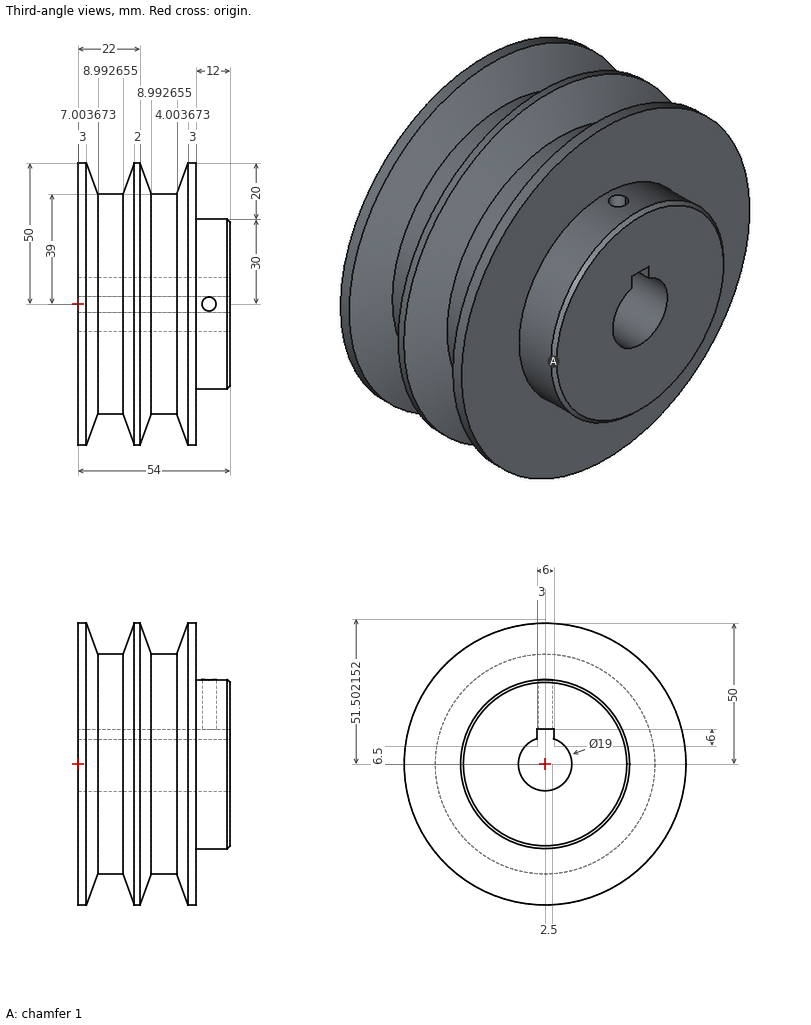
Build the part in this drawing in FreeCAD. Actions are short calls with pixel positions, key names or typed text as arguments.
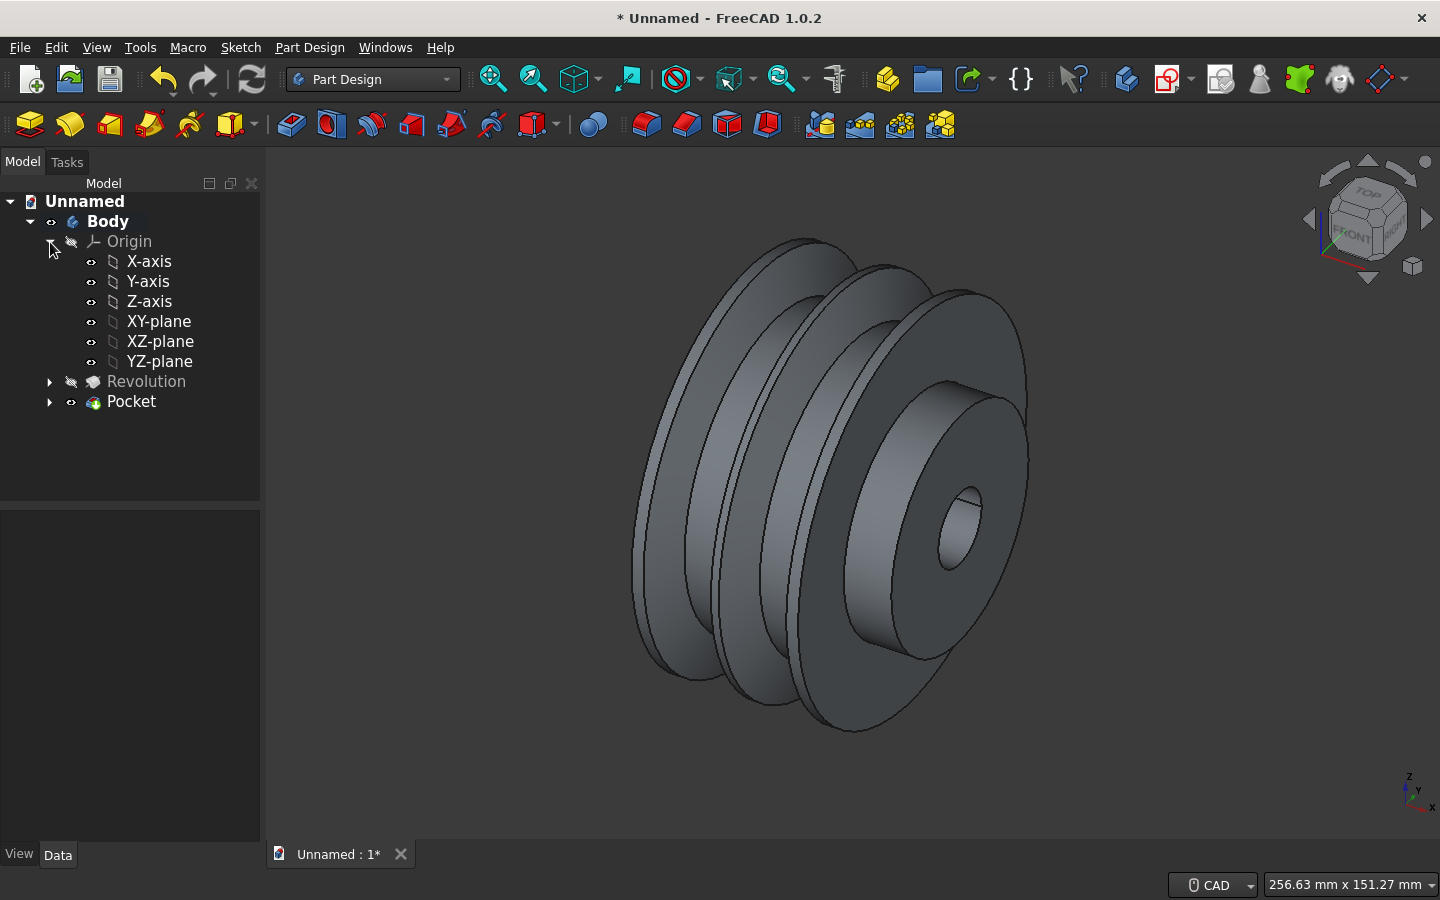
click(136, 362)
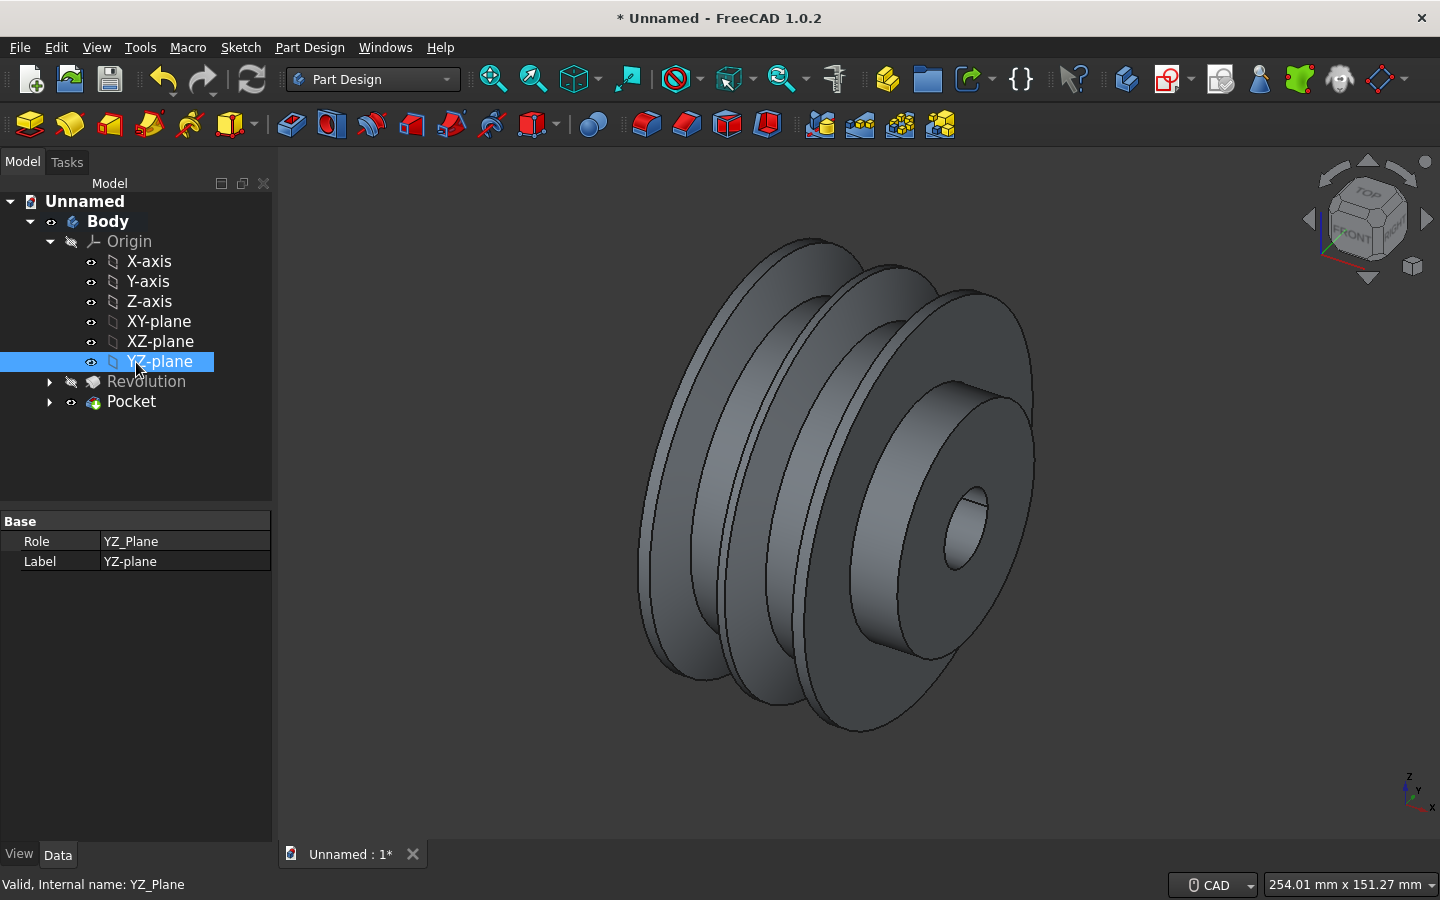
click(1380, 80)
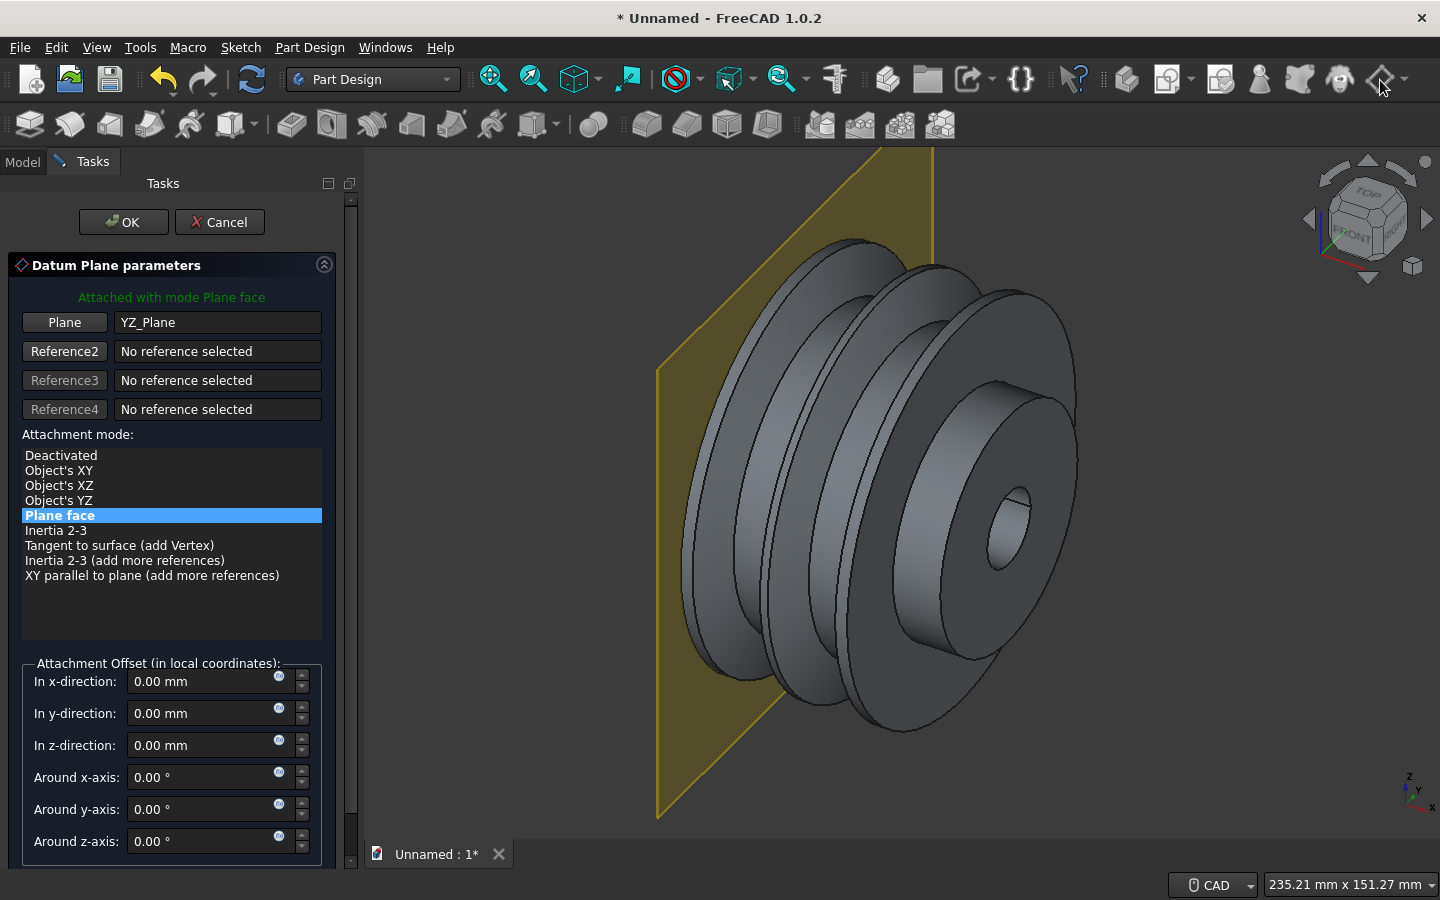
triple_click(210, 745)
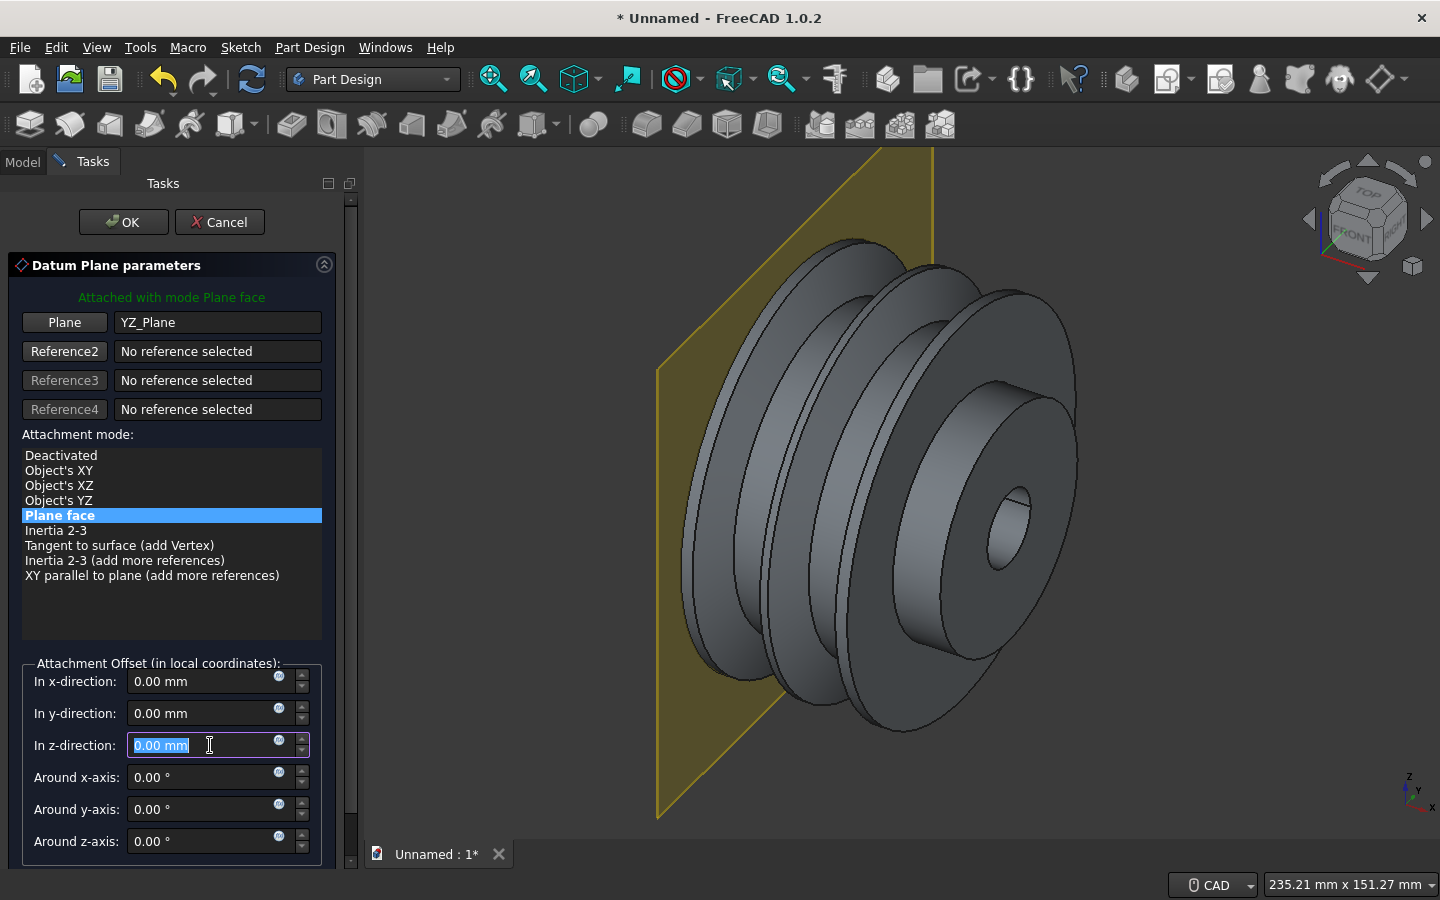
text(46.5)
key(Tab)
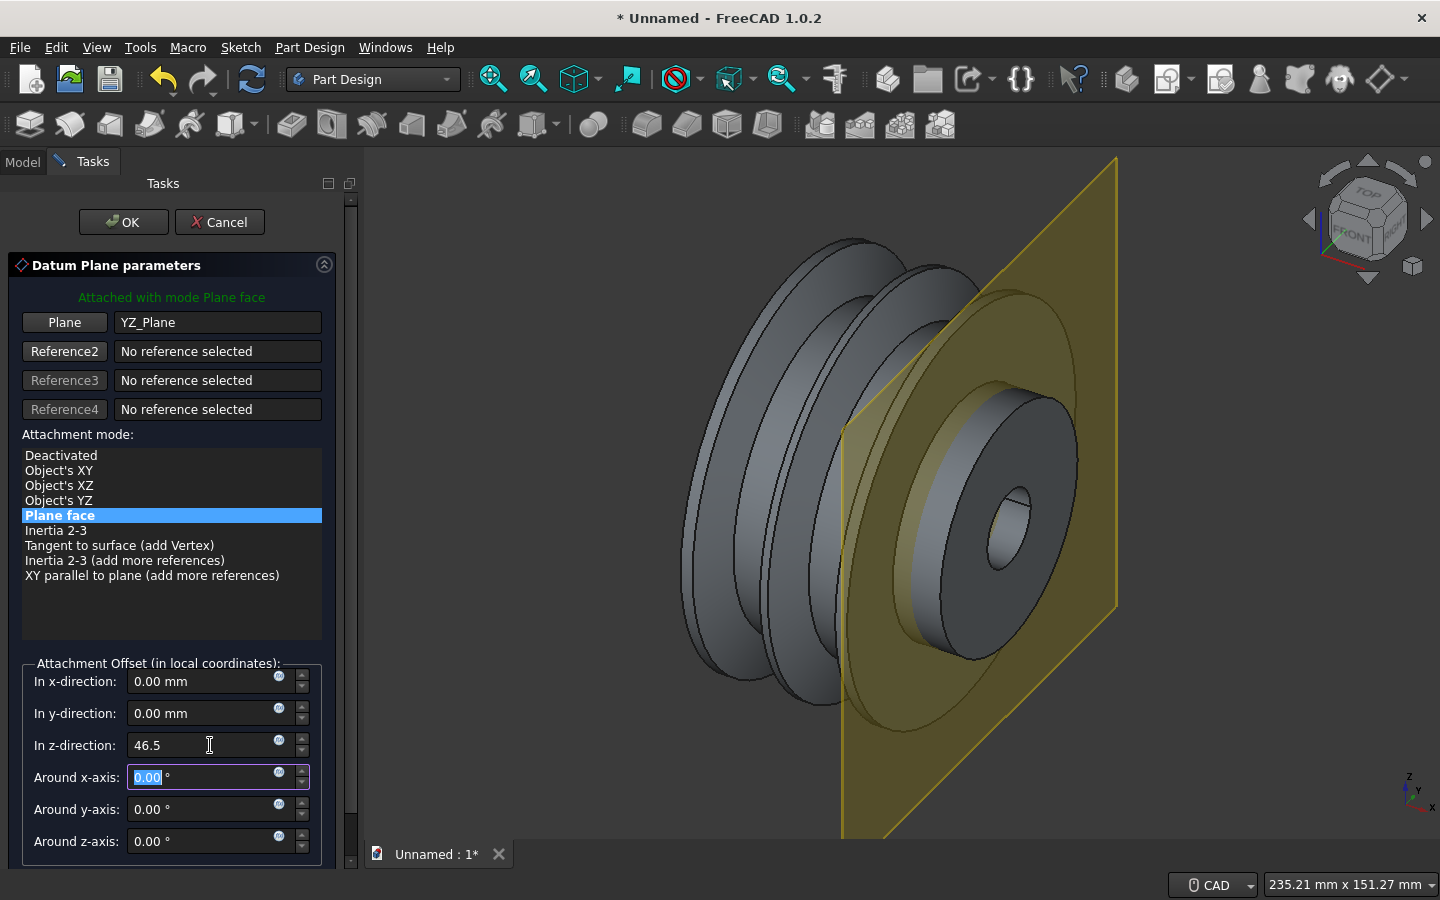
click(124, 222)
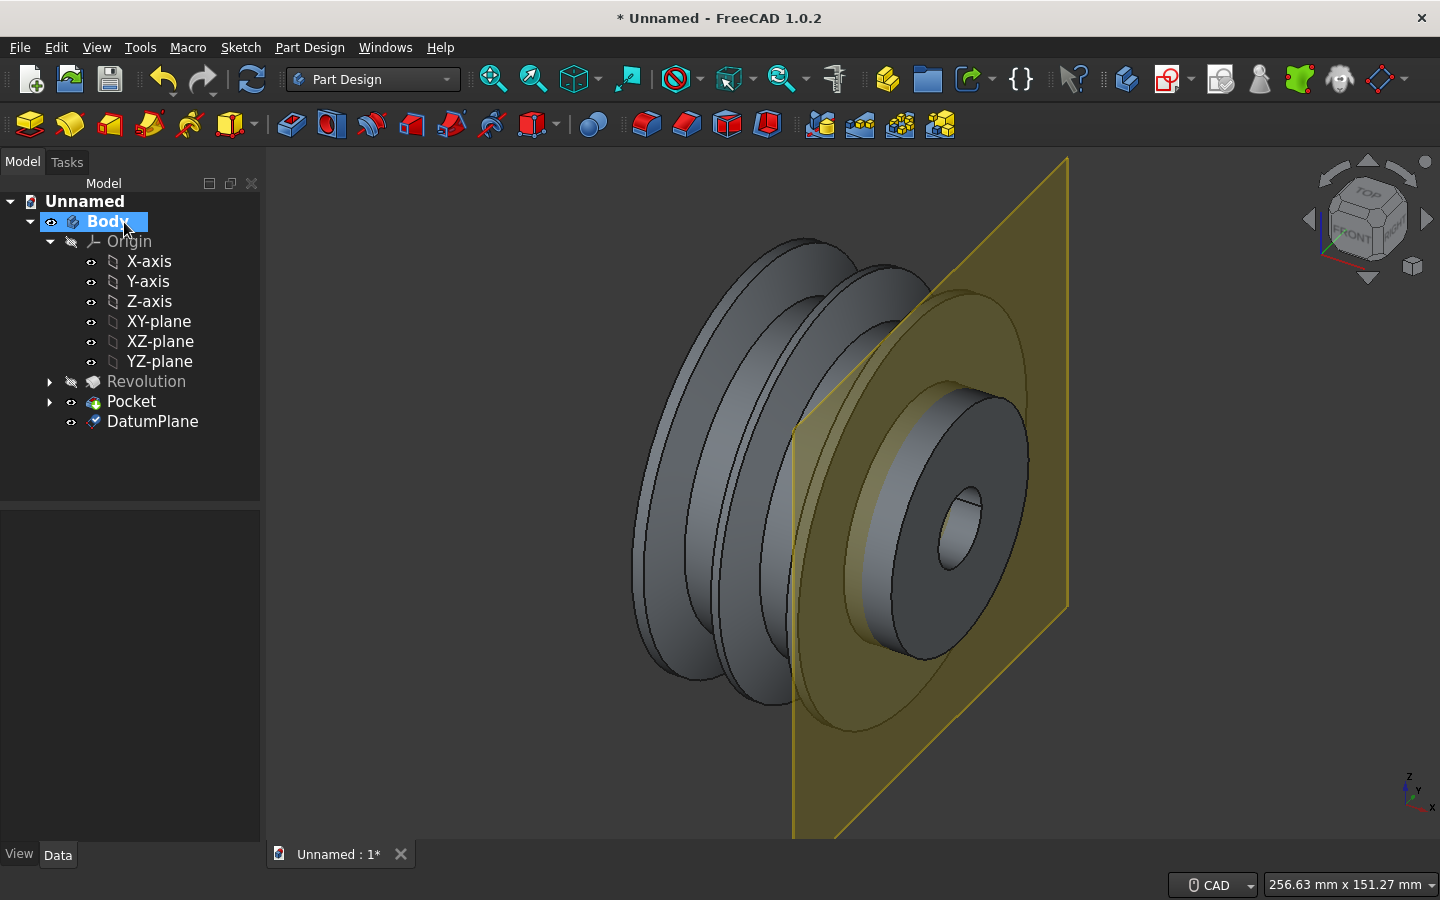
click(116, 422)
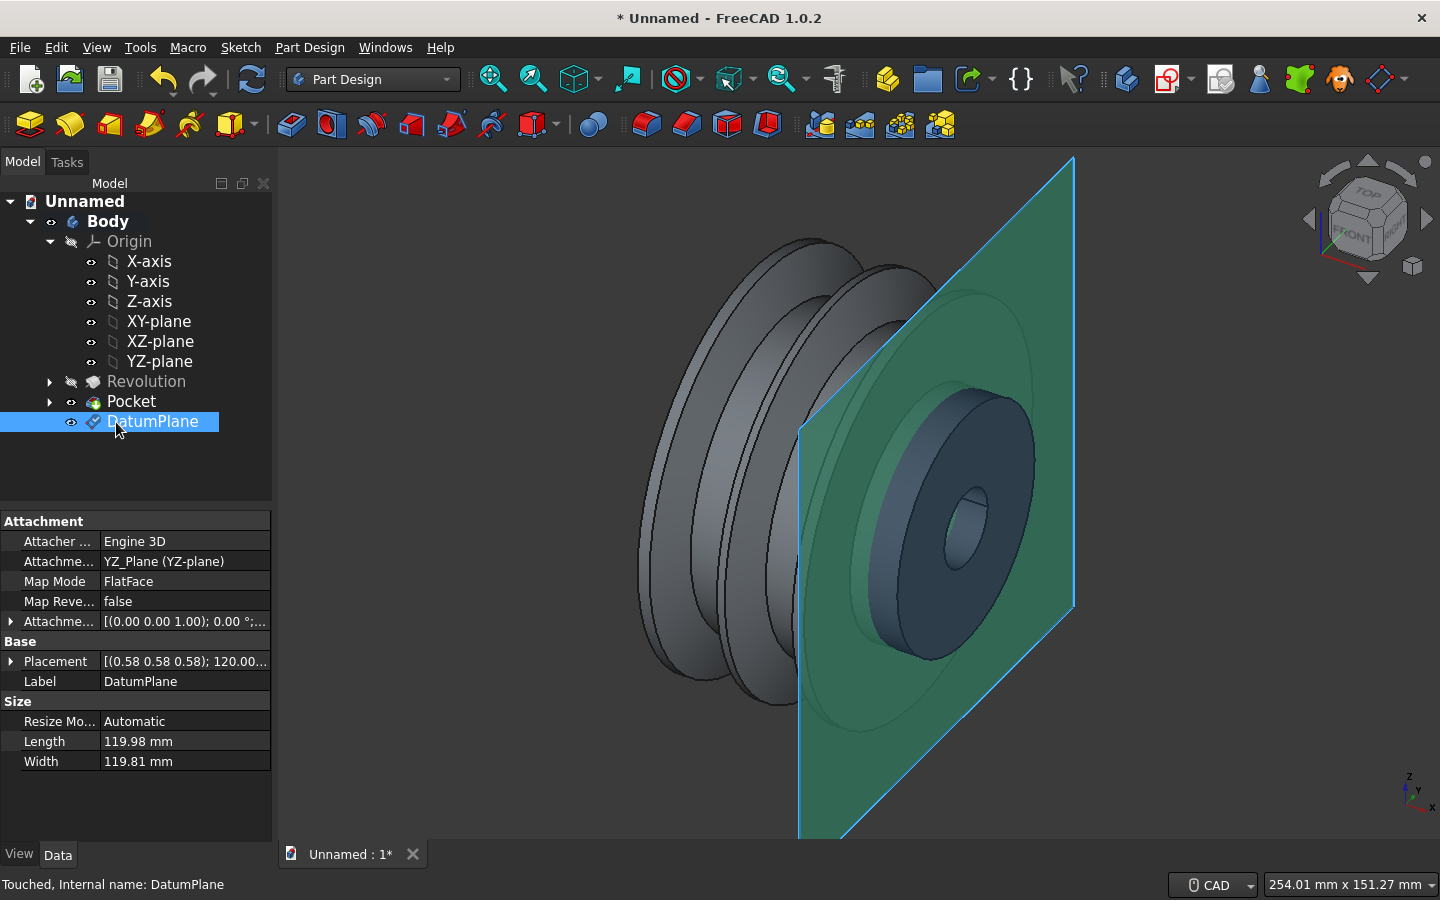
click(1168, 80)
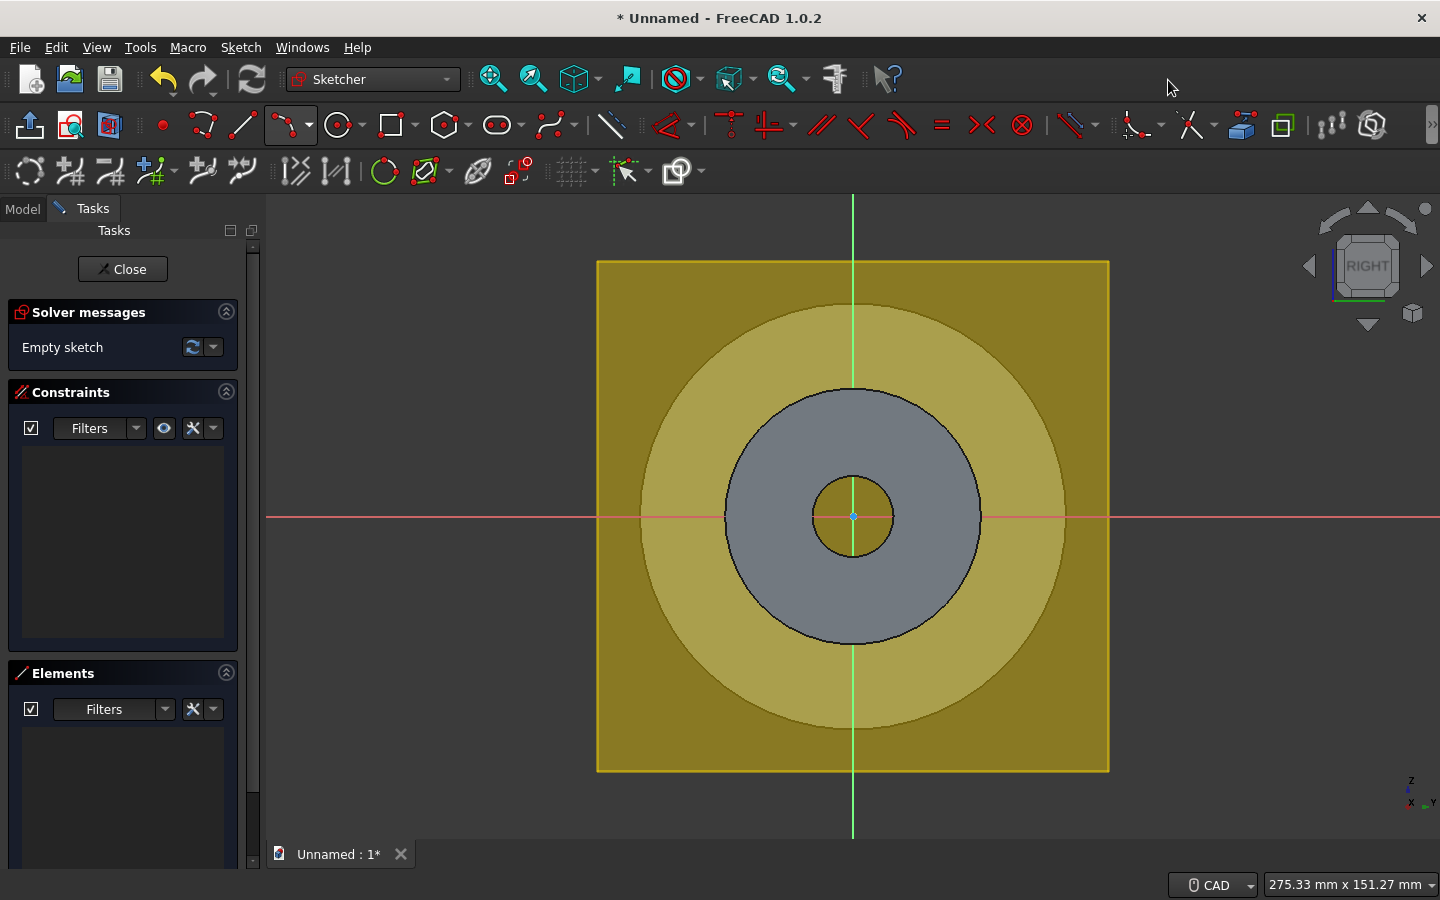
click(110, 126)